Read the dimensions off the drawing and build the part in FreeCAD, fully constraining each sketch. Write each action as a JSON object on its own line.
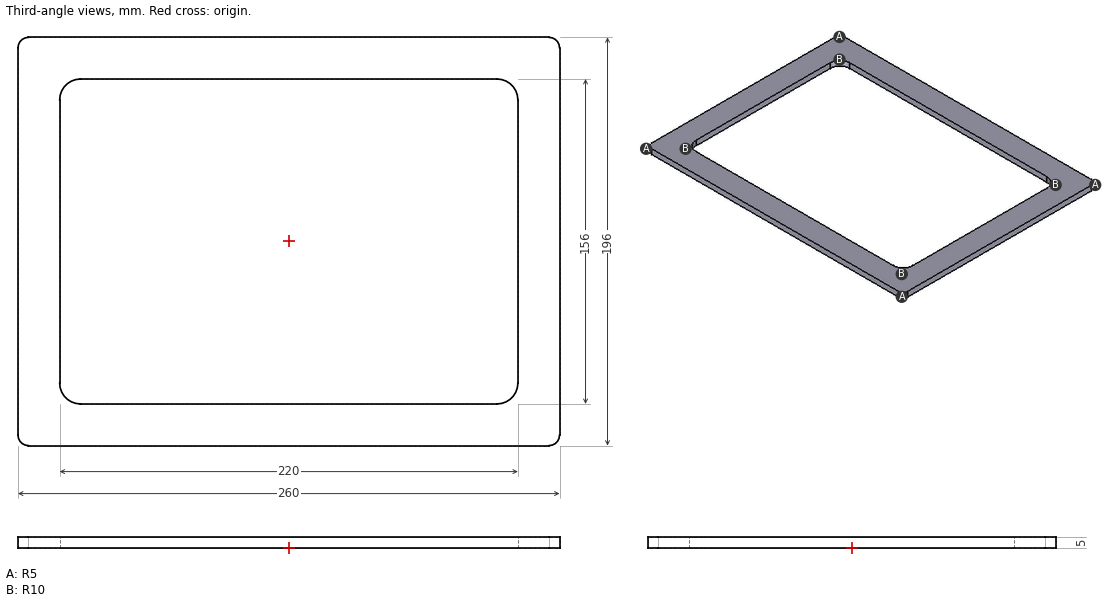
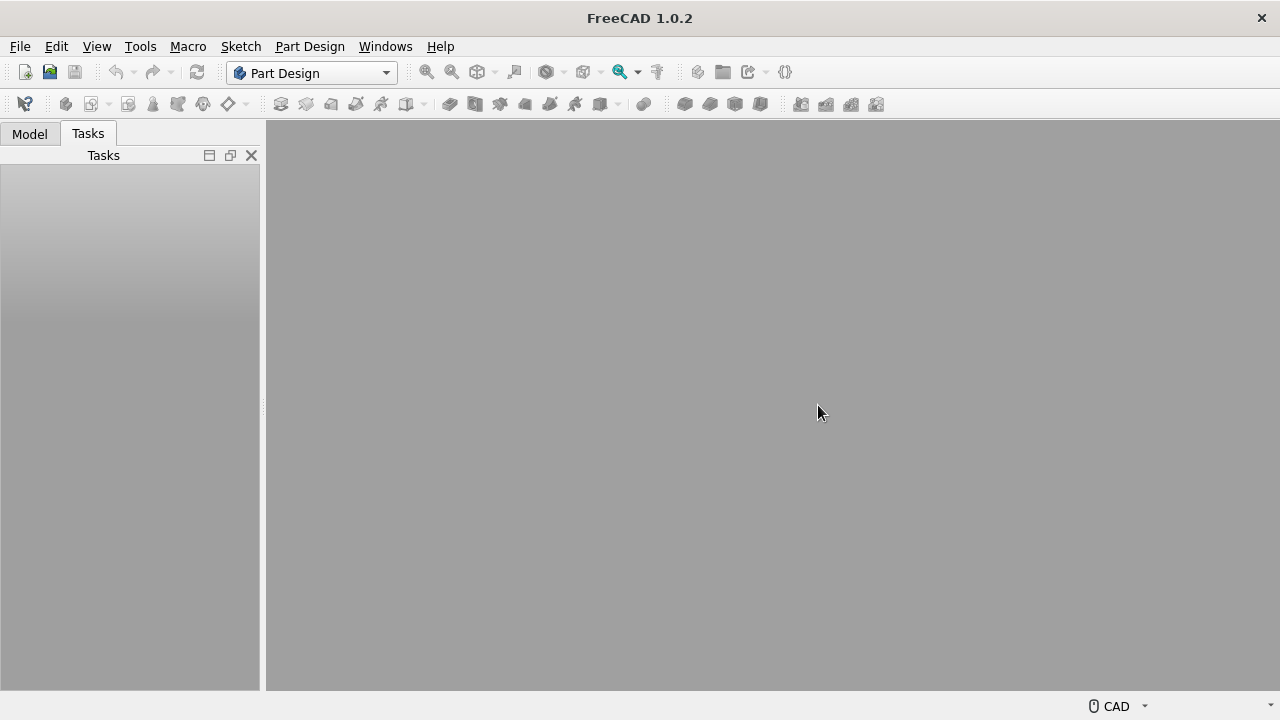
{"action": "left_click", "coordinate": [25, 72]}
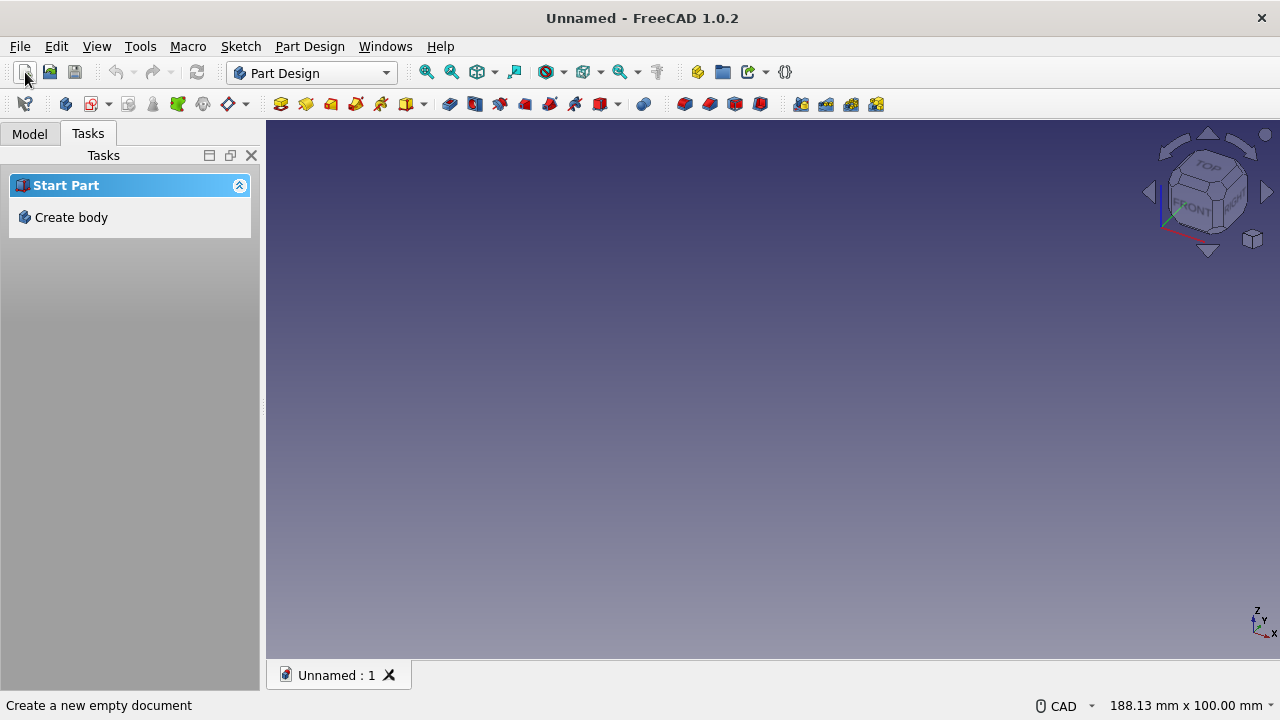
{"action": "left_click", "coordinate": [90, 104]}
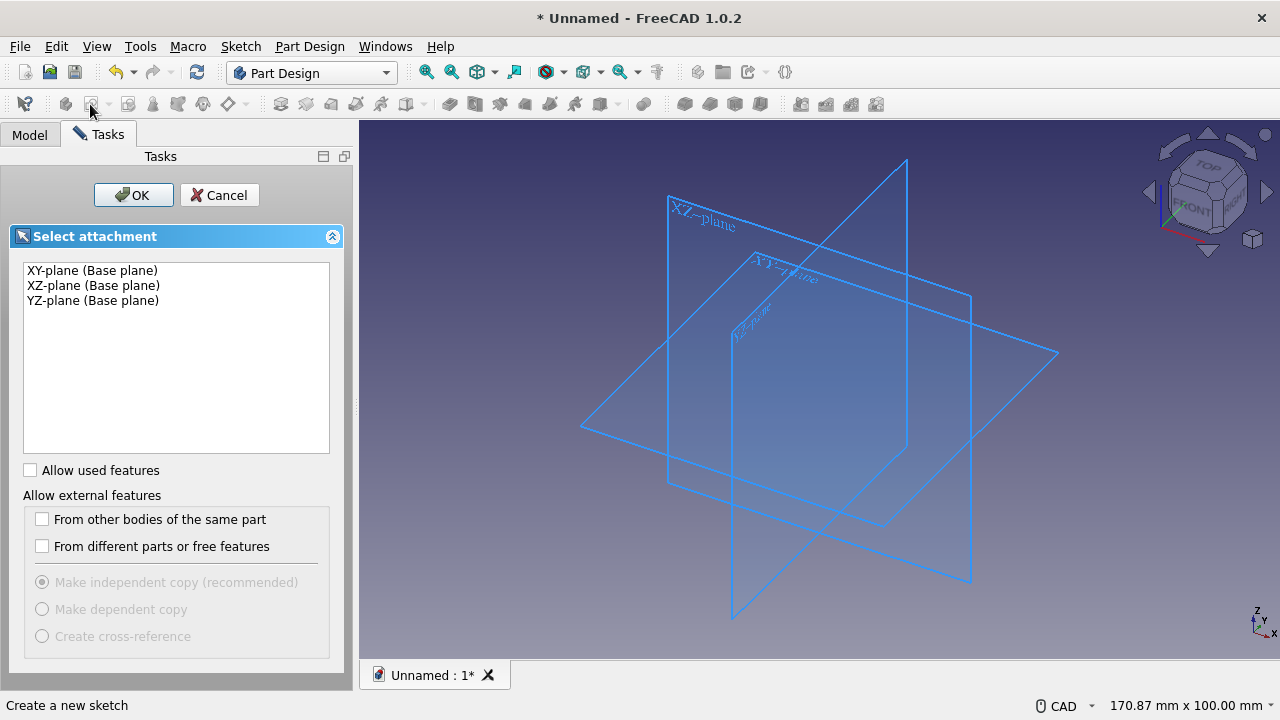
{"action": "left_click", "coordinate": [84, 270]}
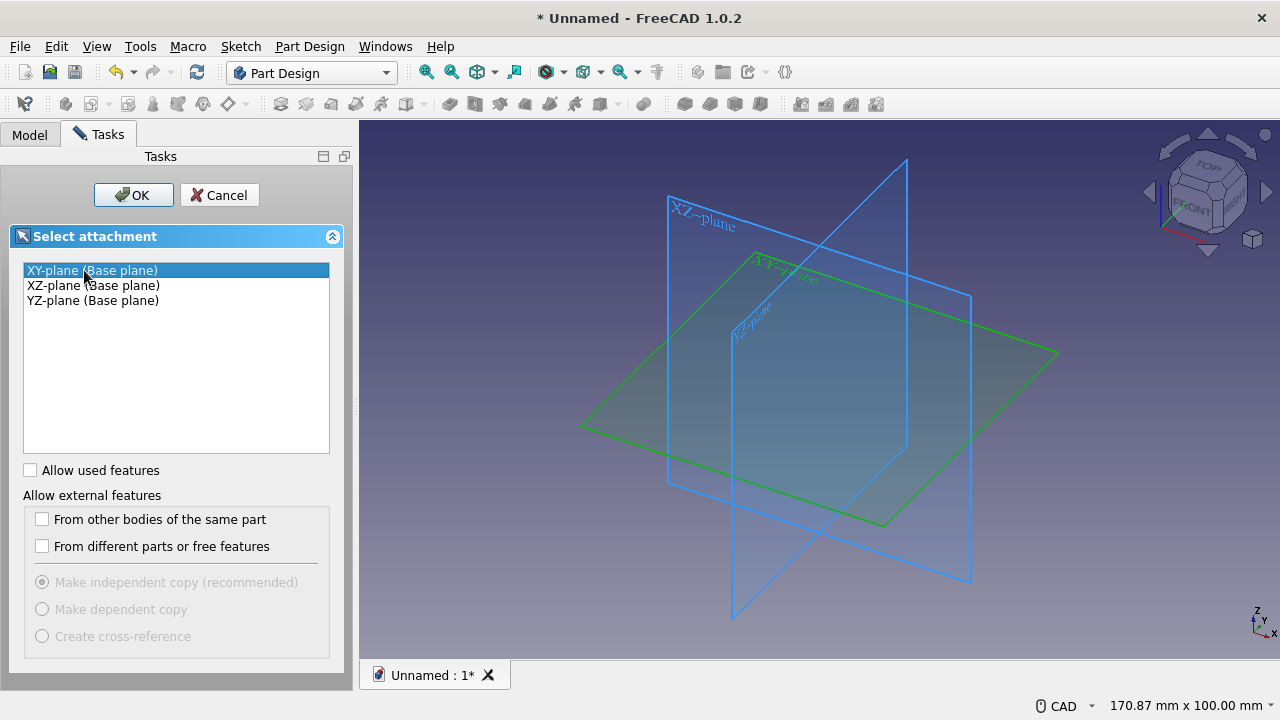
{"action": "left_click", "coordinate": [134, 195]}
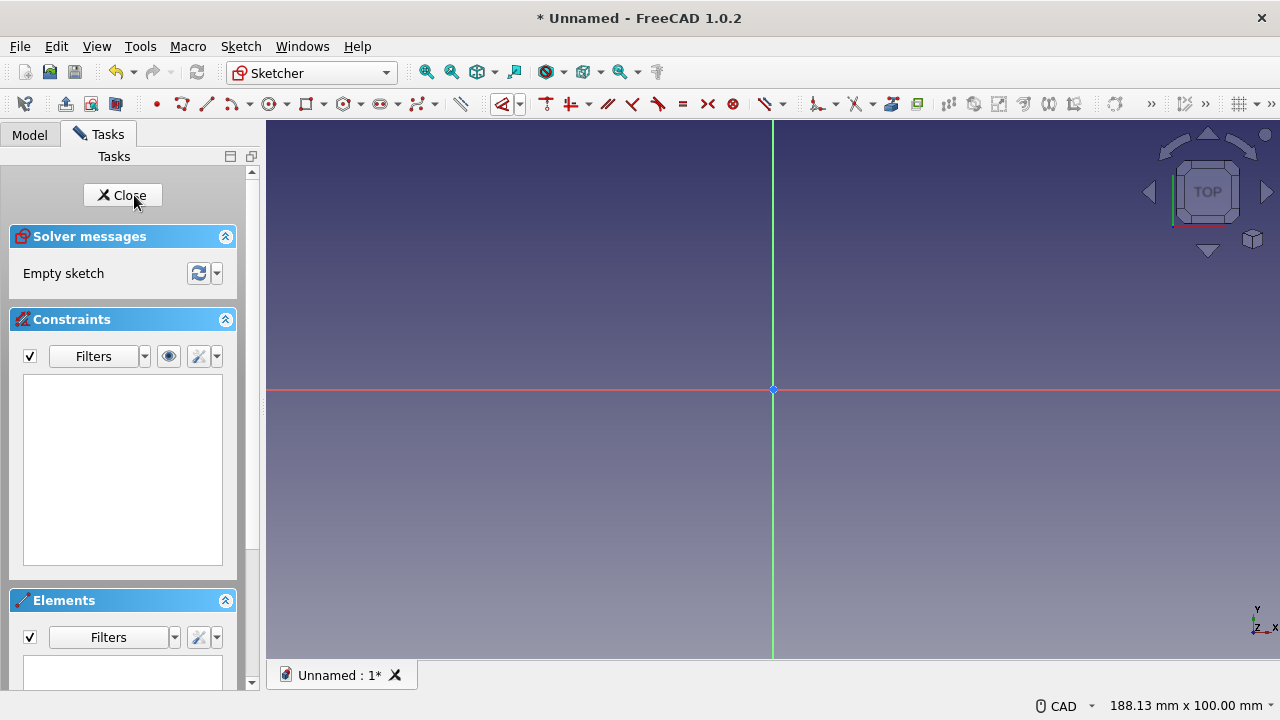
{"action": "scroll", "coordinate": [675, 389], "scroll_direction": "down", "scroll_amount": 6}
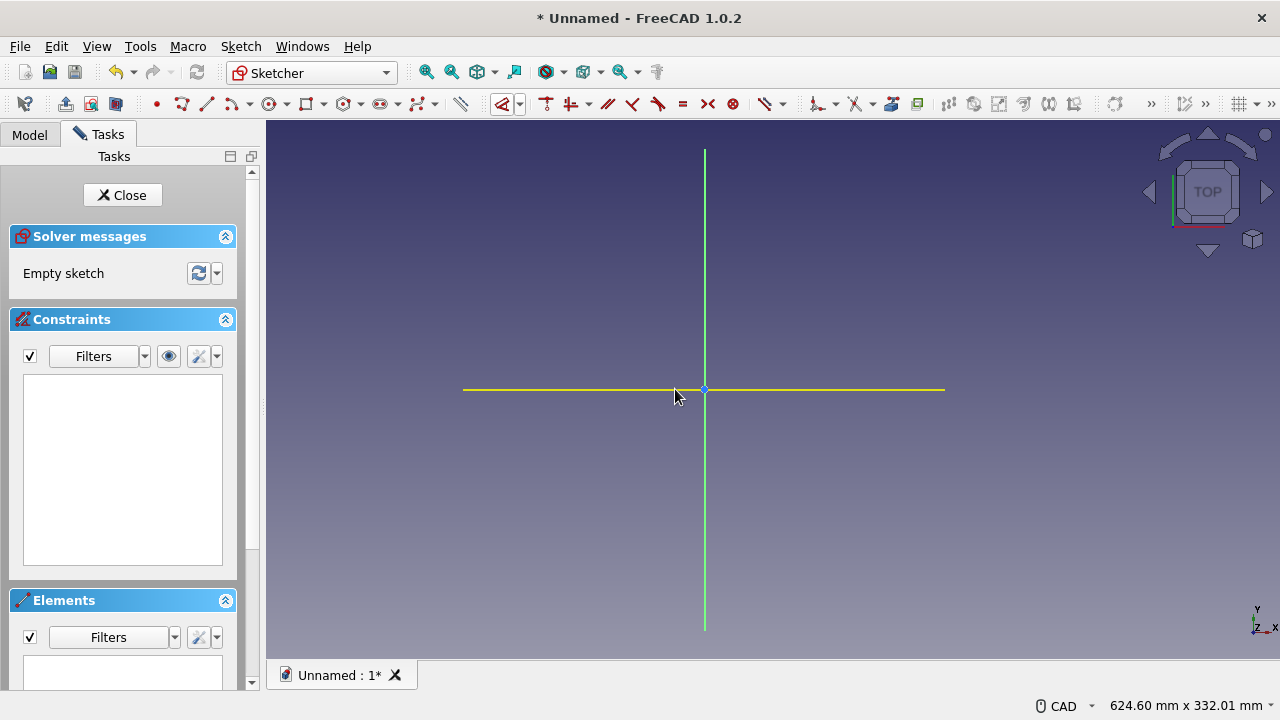
{"action": "key", "text": "g v"}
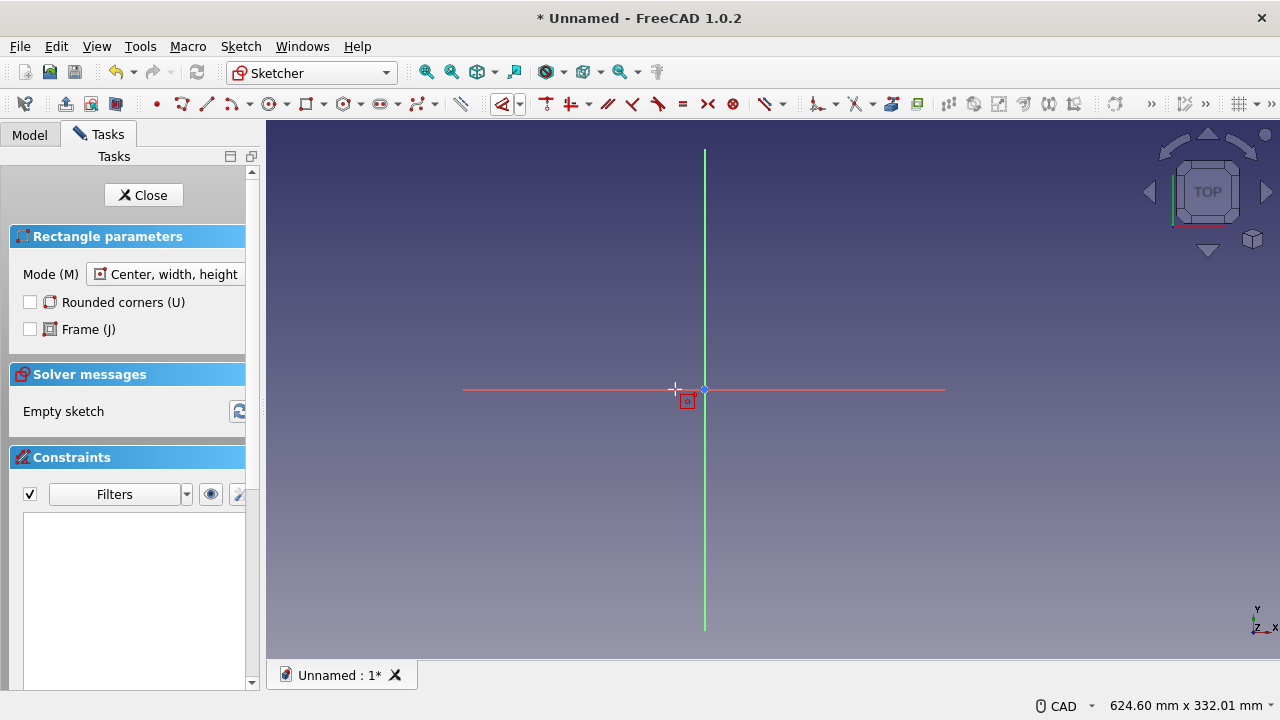
{"action": "left_click", "coordinate": [705, 390]}
{"action": "left_click", "coordinate": [916, 230]}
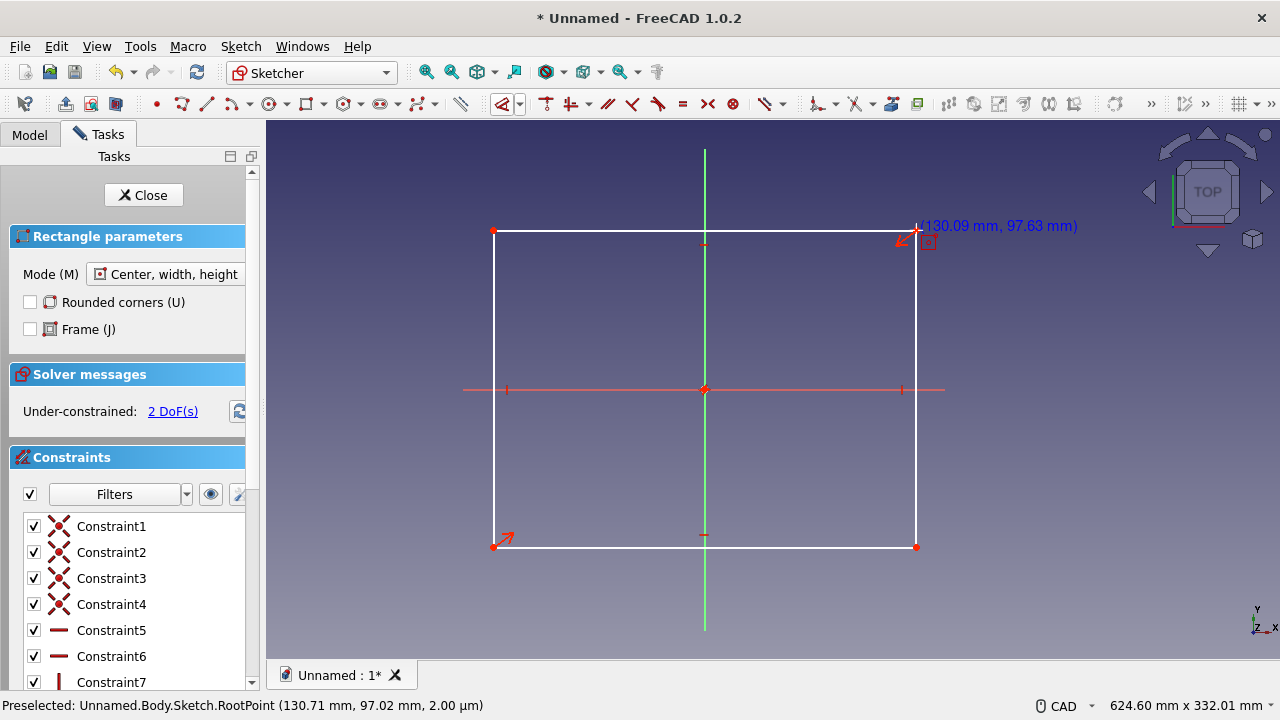
{"action": "left_click", "coordinate": [705, 390]}
{"action": "left_click", "coordinate": [883, 263]}
{"action": "key", "text": "Escape"}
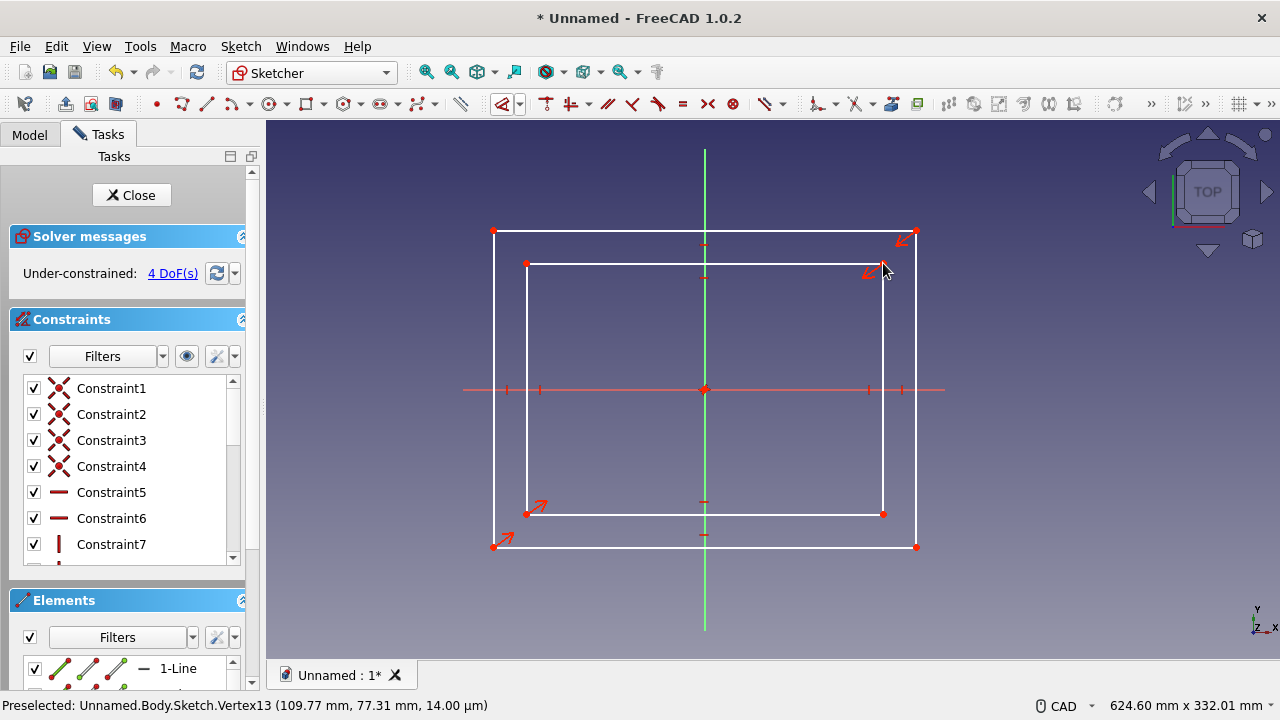
{"action": "left_click", "coordinate": [502, 104]}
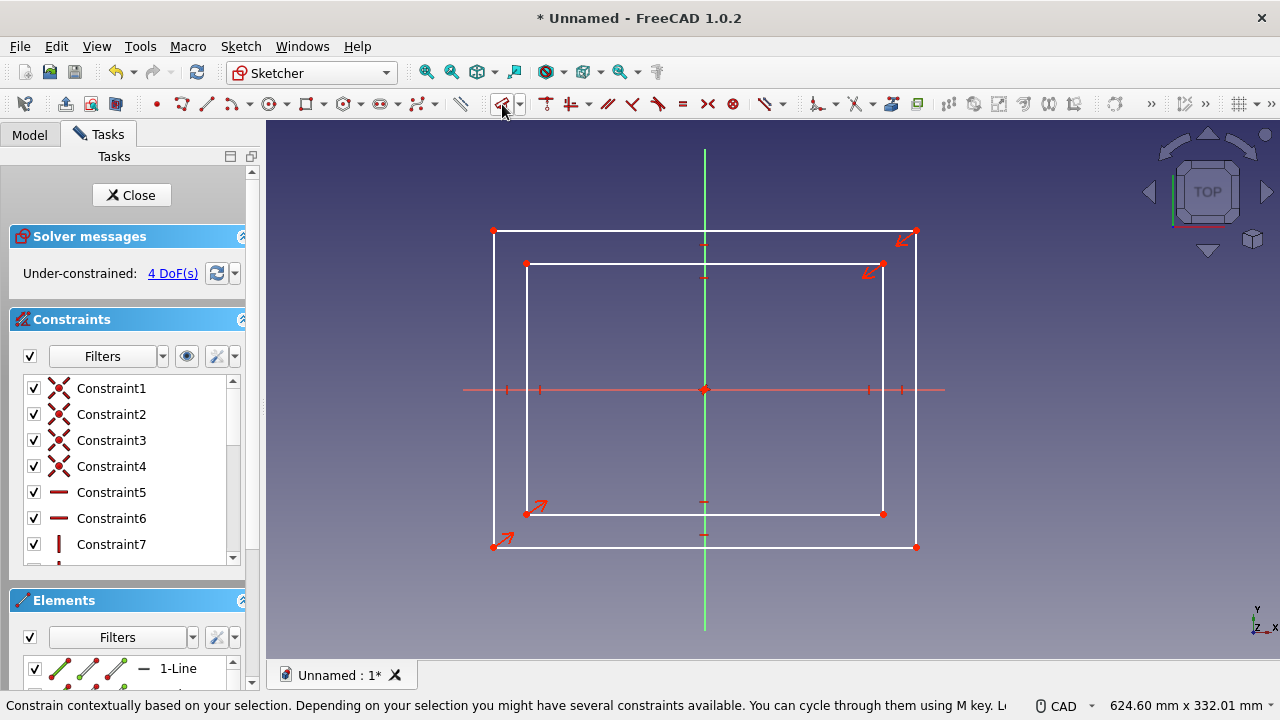
{"action": "left_click", "coordinate": [620, 548]}
{"action": "left_click", "coordinate": [608, 582]}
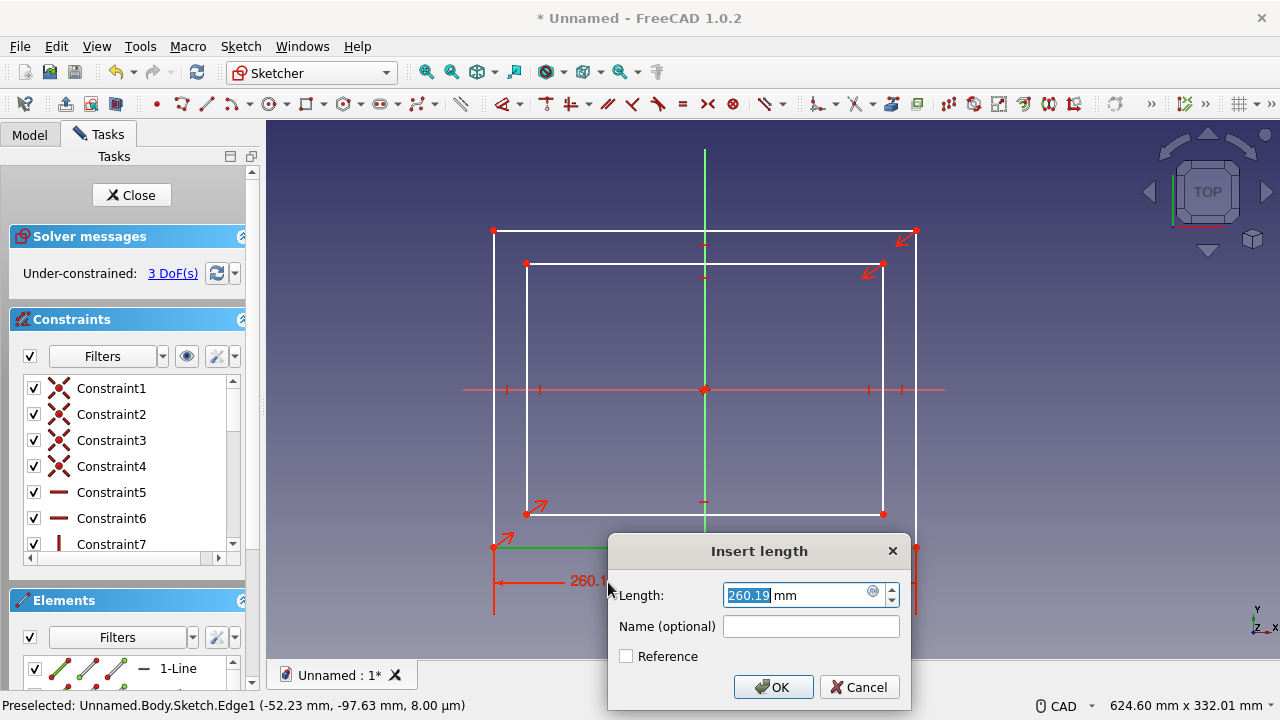
{"action": "type", "text": "260"}
{"action": "key", "text": "Return"}